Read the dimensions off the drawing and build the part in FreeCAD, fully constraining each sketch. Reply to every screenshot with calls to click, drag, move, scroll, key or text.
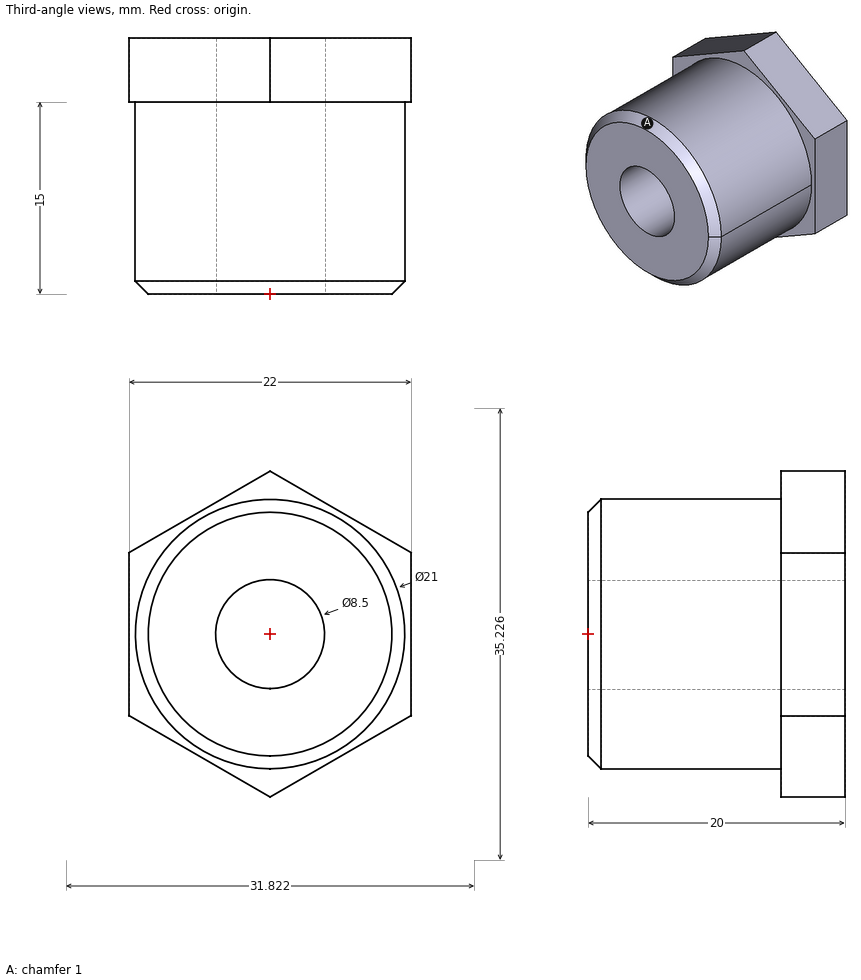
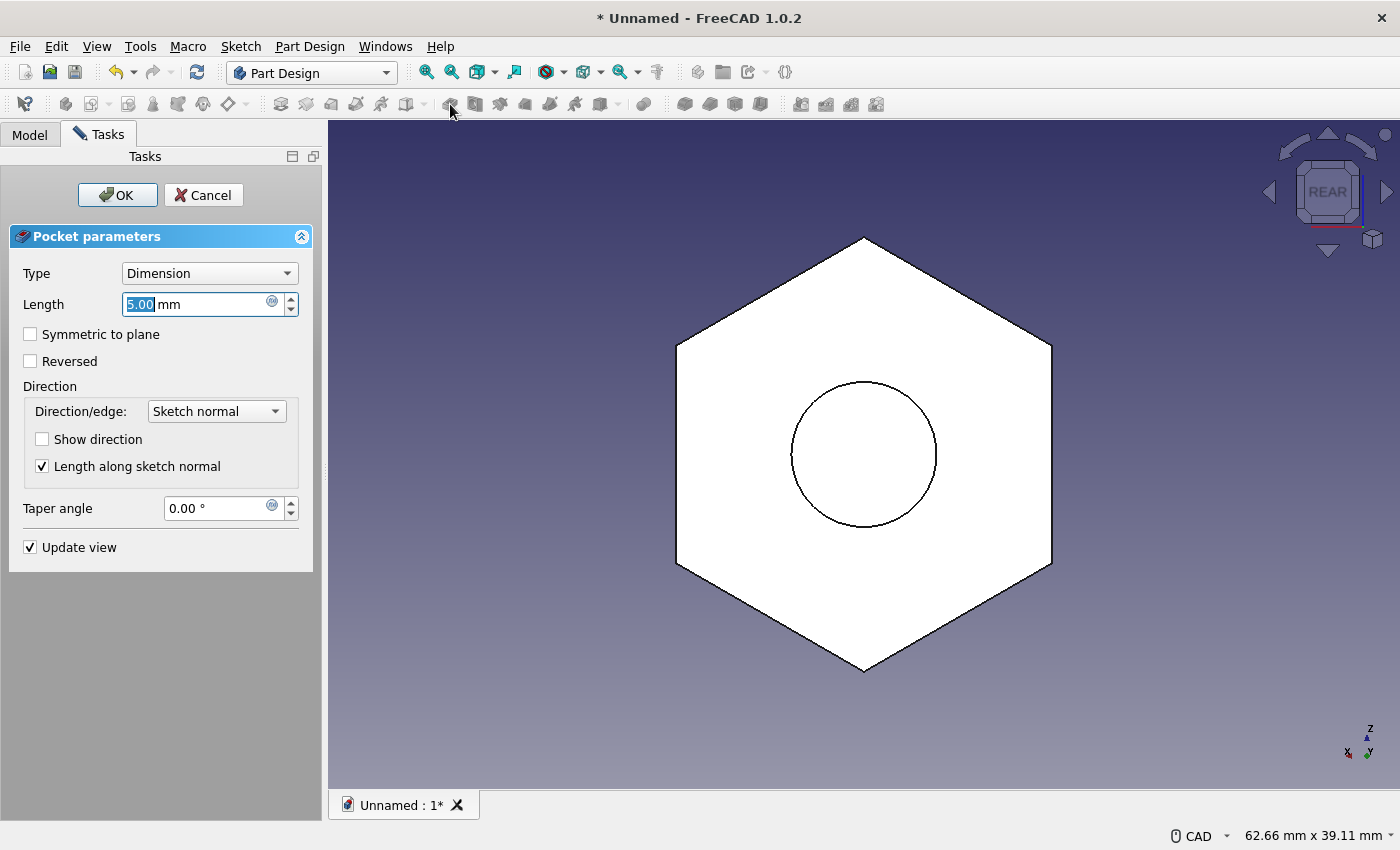
click(210, 274)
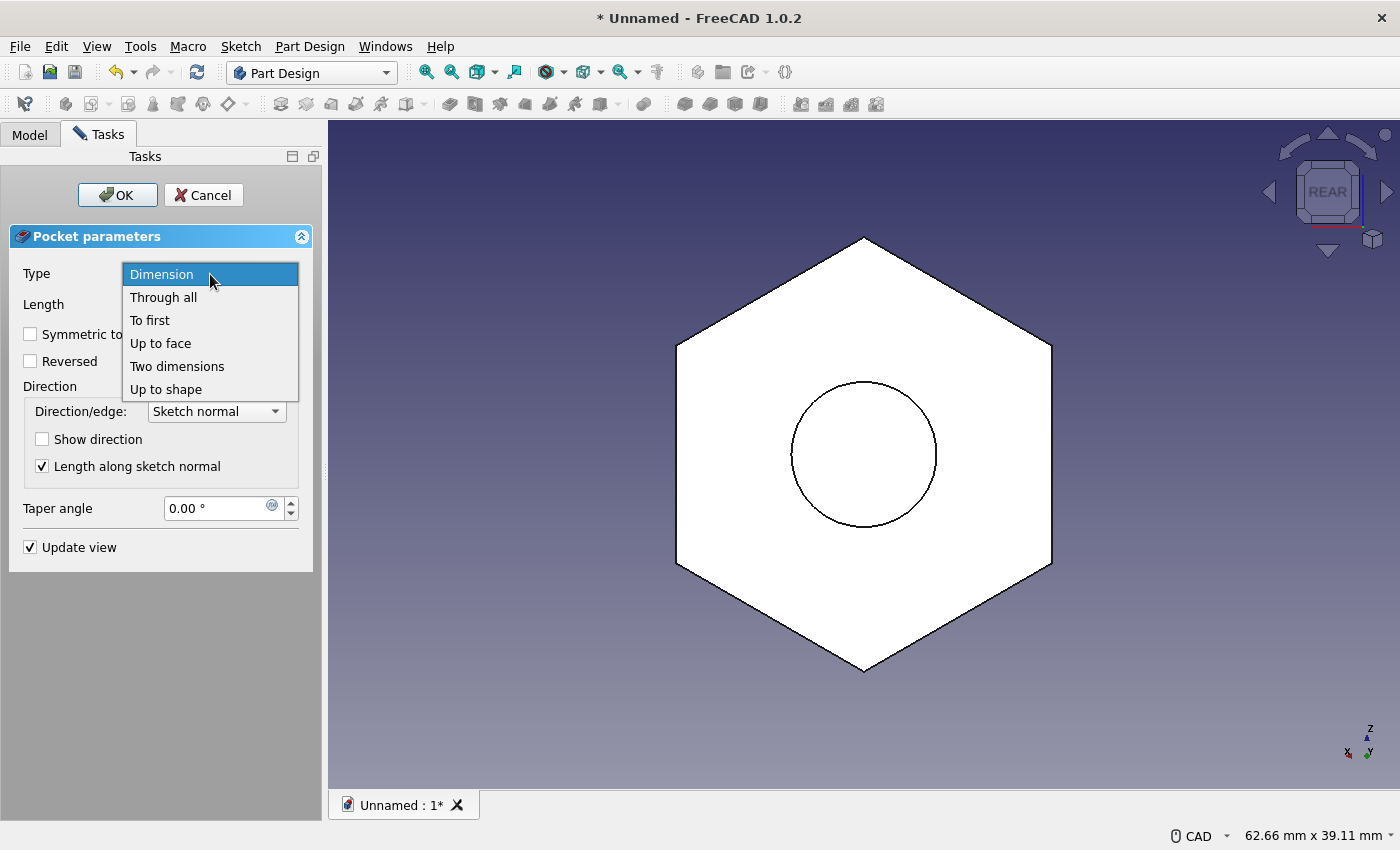
click(208, 298)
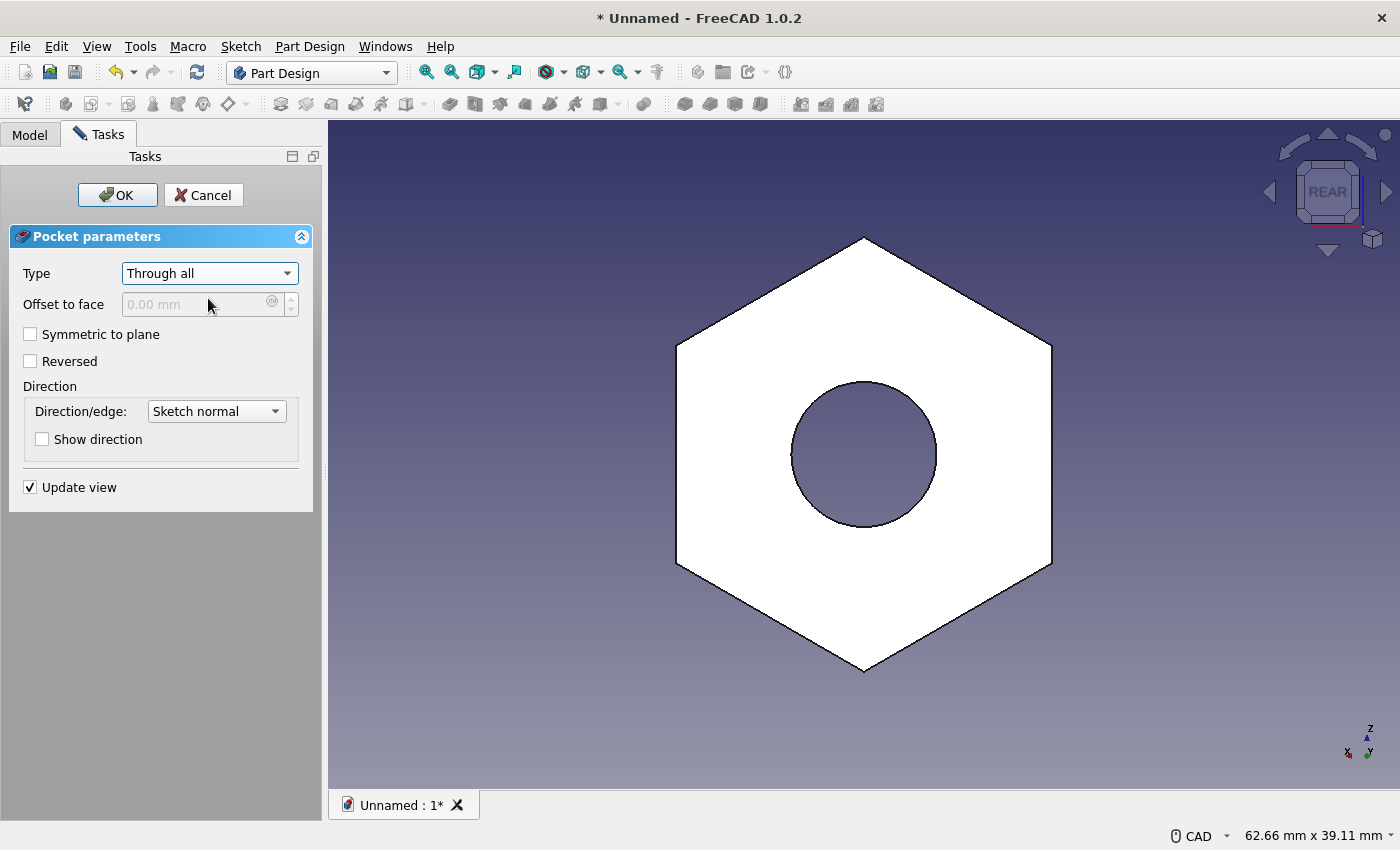
click(118, 195)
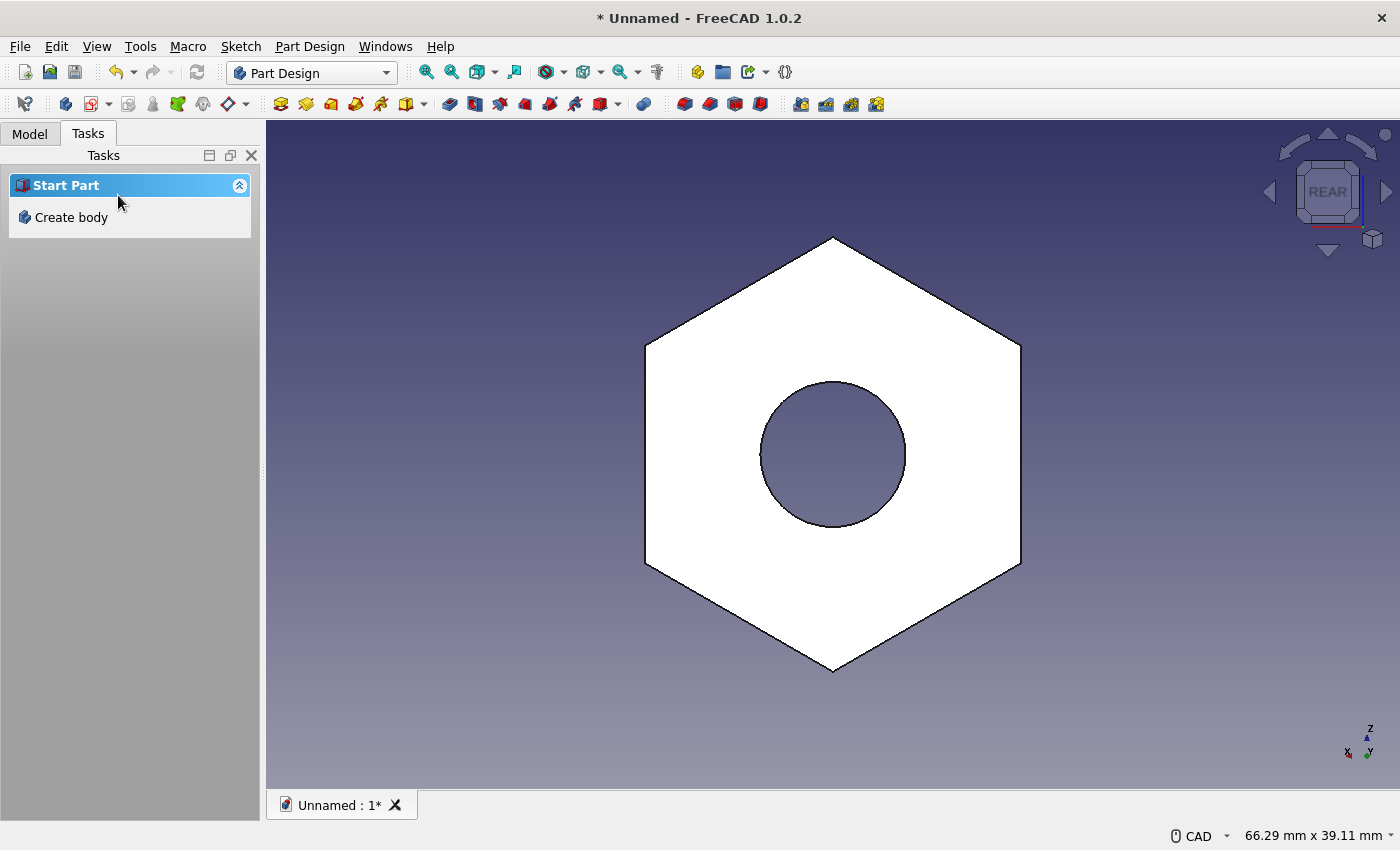
key(0)